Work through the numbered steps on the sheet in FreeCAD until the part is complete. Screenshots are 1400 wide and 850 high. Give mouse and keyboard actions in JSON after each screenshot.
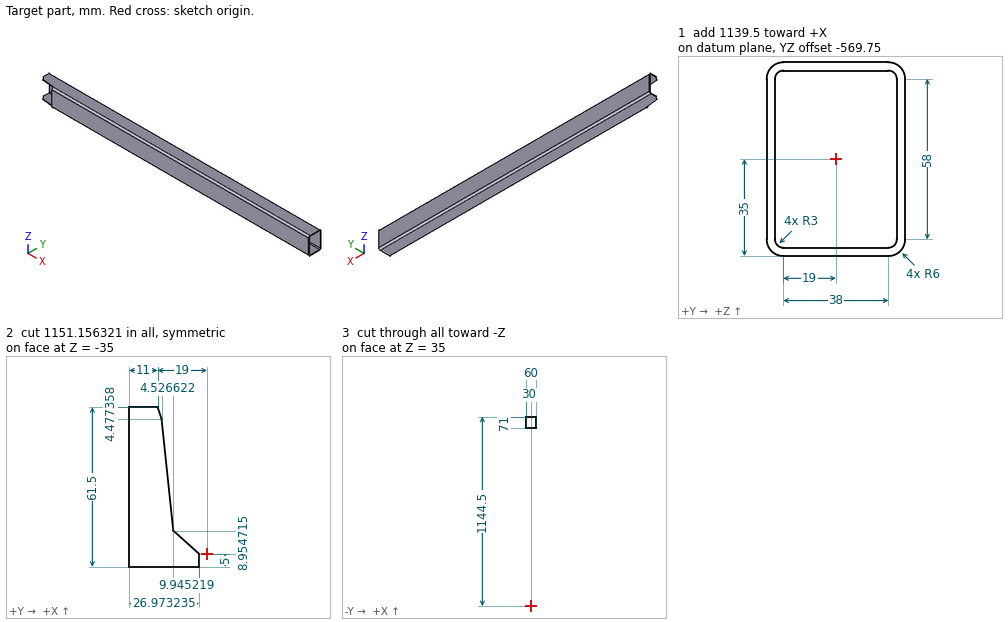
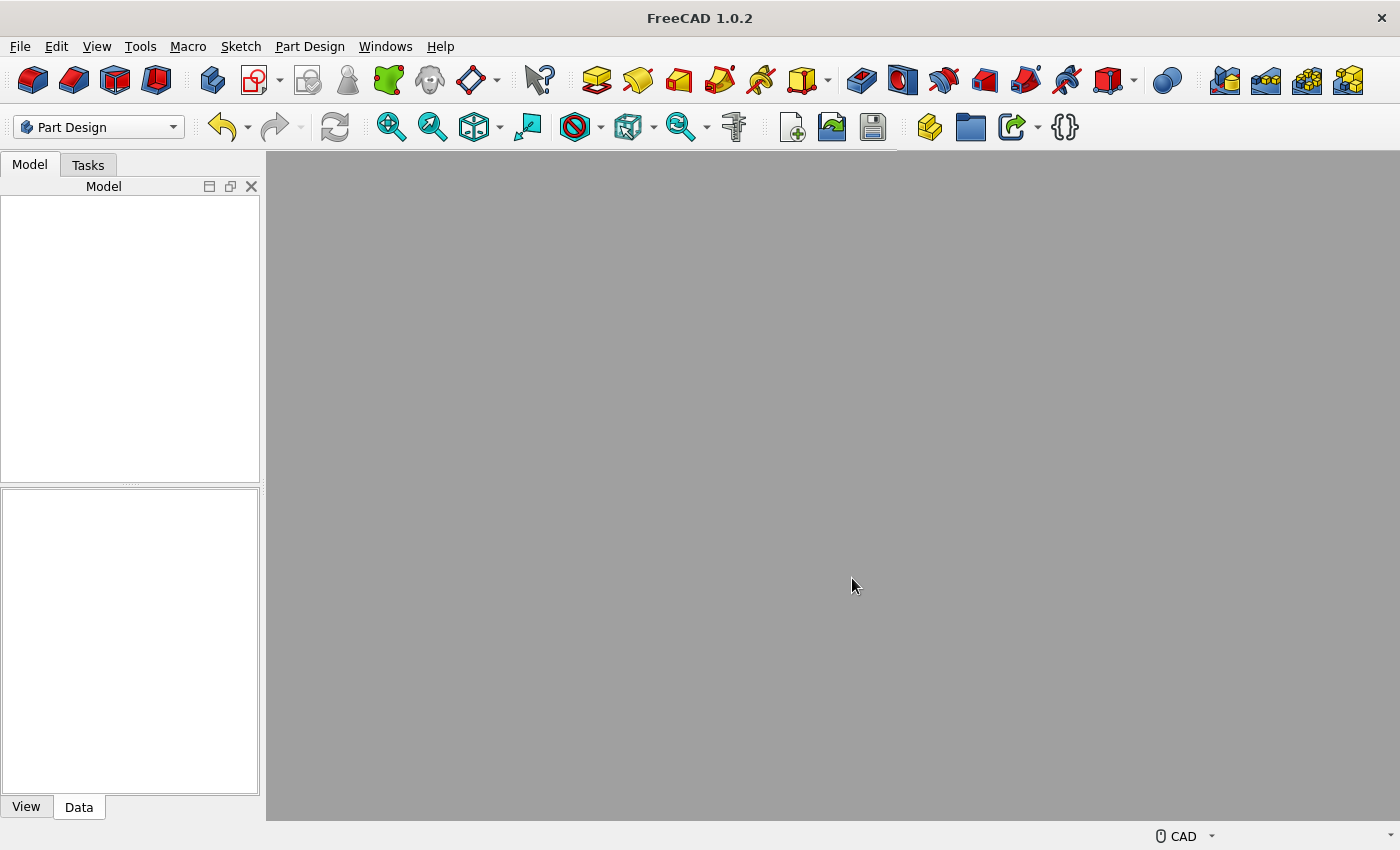
{"action": "key", "text": "ctrl+n"}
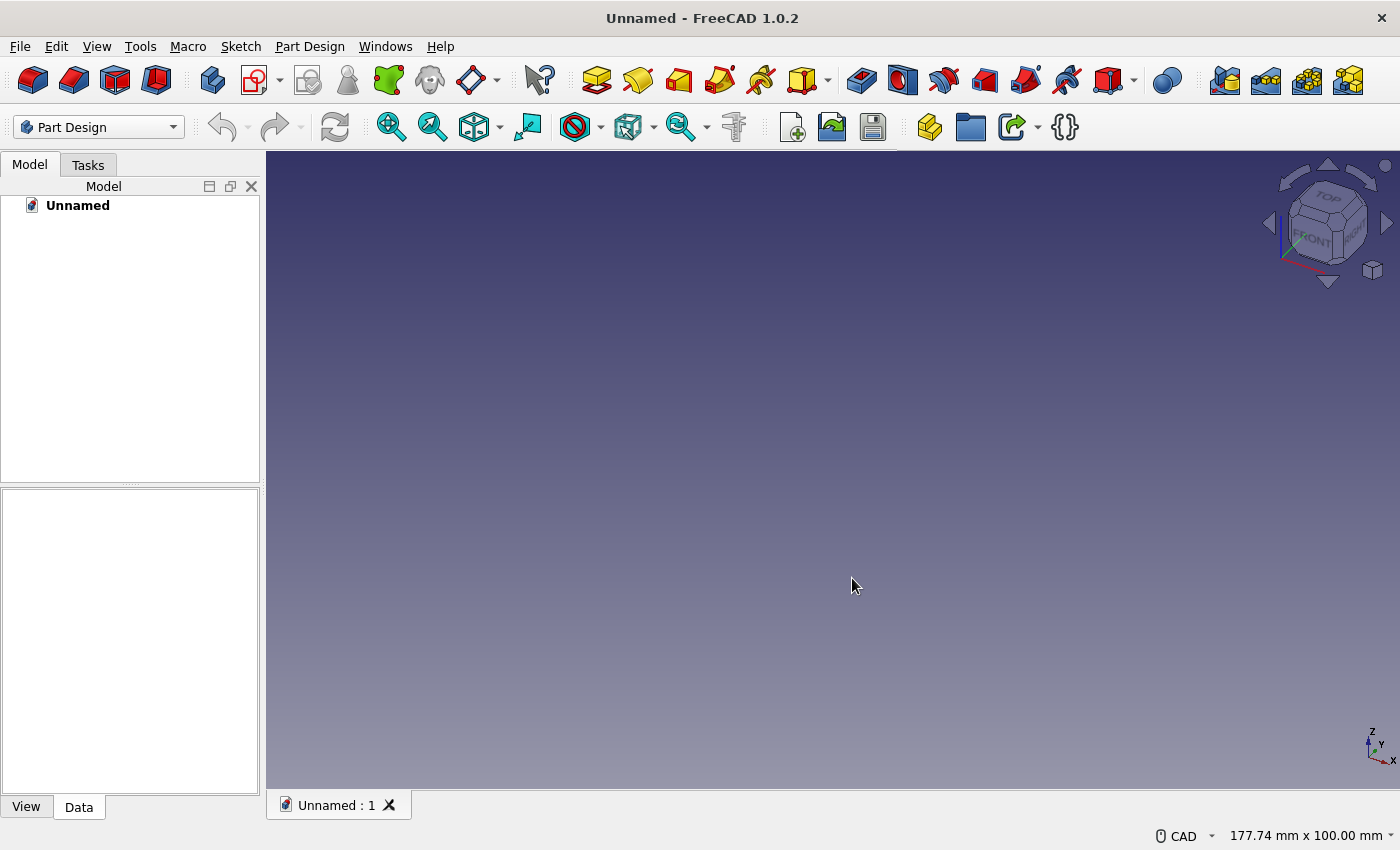
{"action": "left_click", "coordinate": [213, 80]}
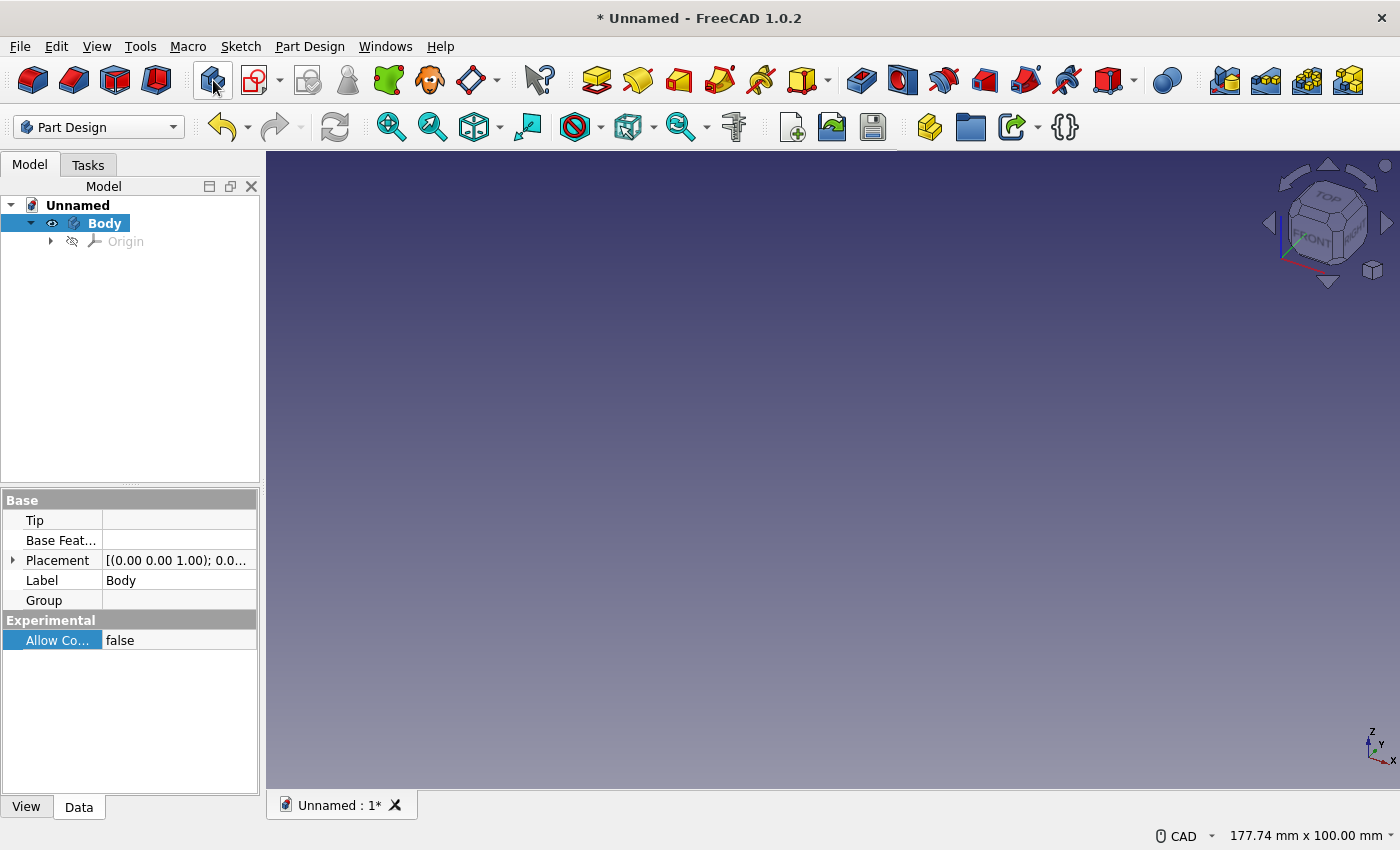
{"action": "left_click", "coordinate": [51, 241]}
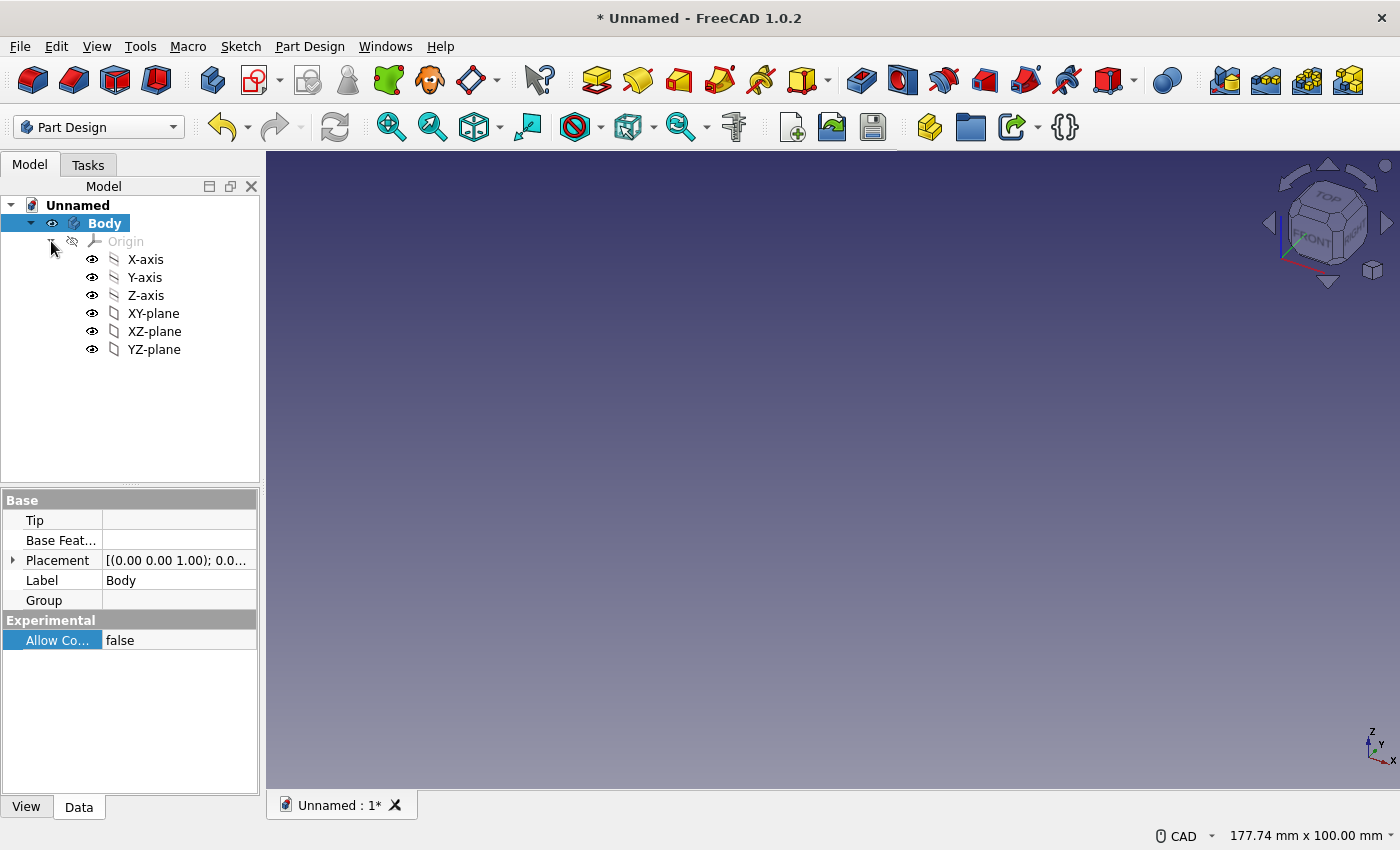
{"action": "left_click", "coordinate": [137, 349]}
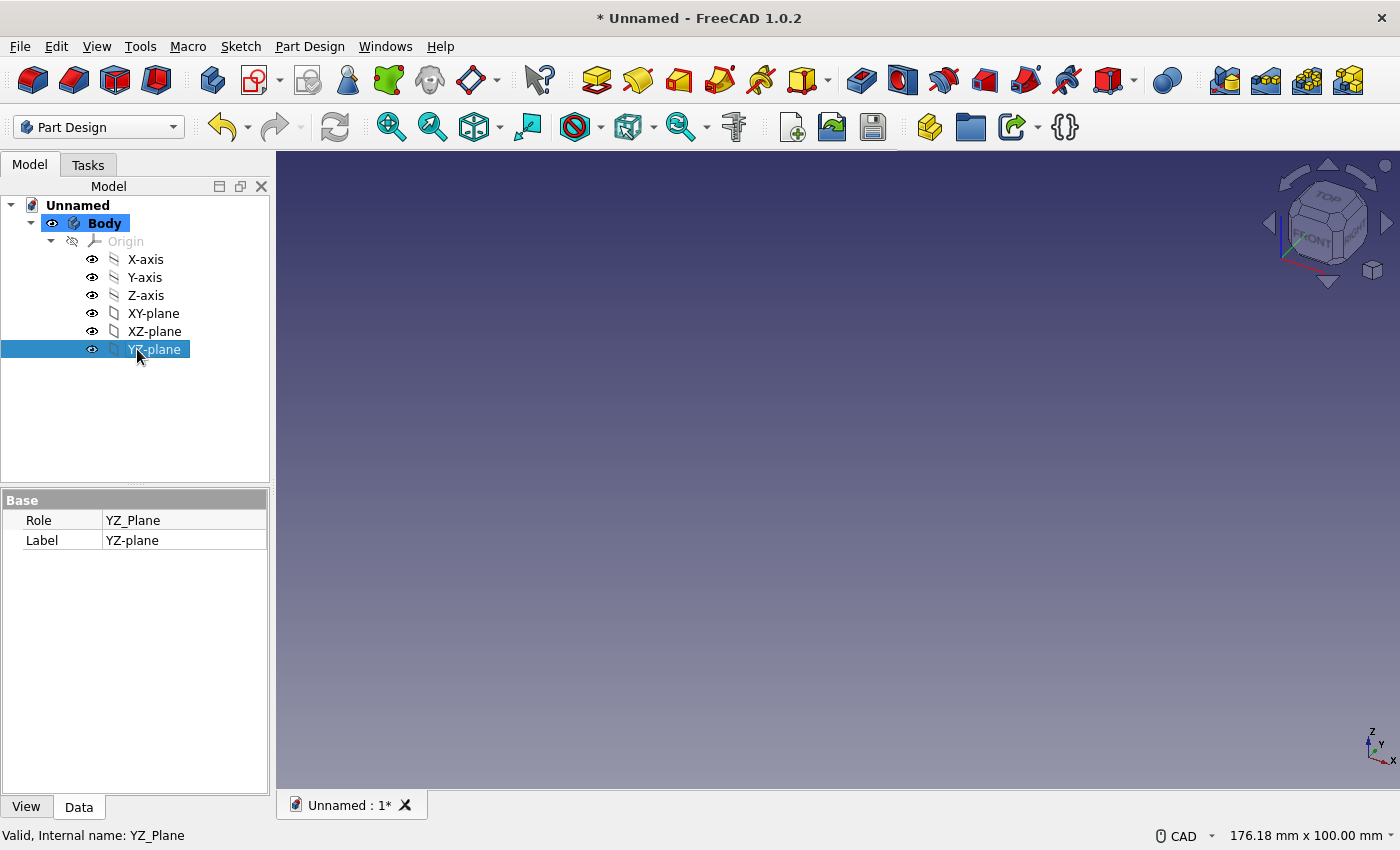
{"action": "left_click", "coordinate": [470, 80]}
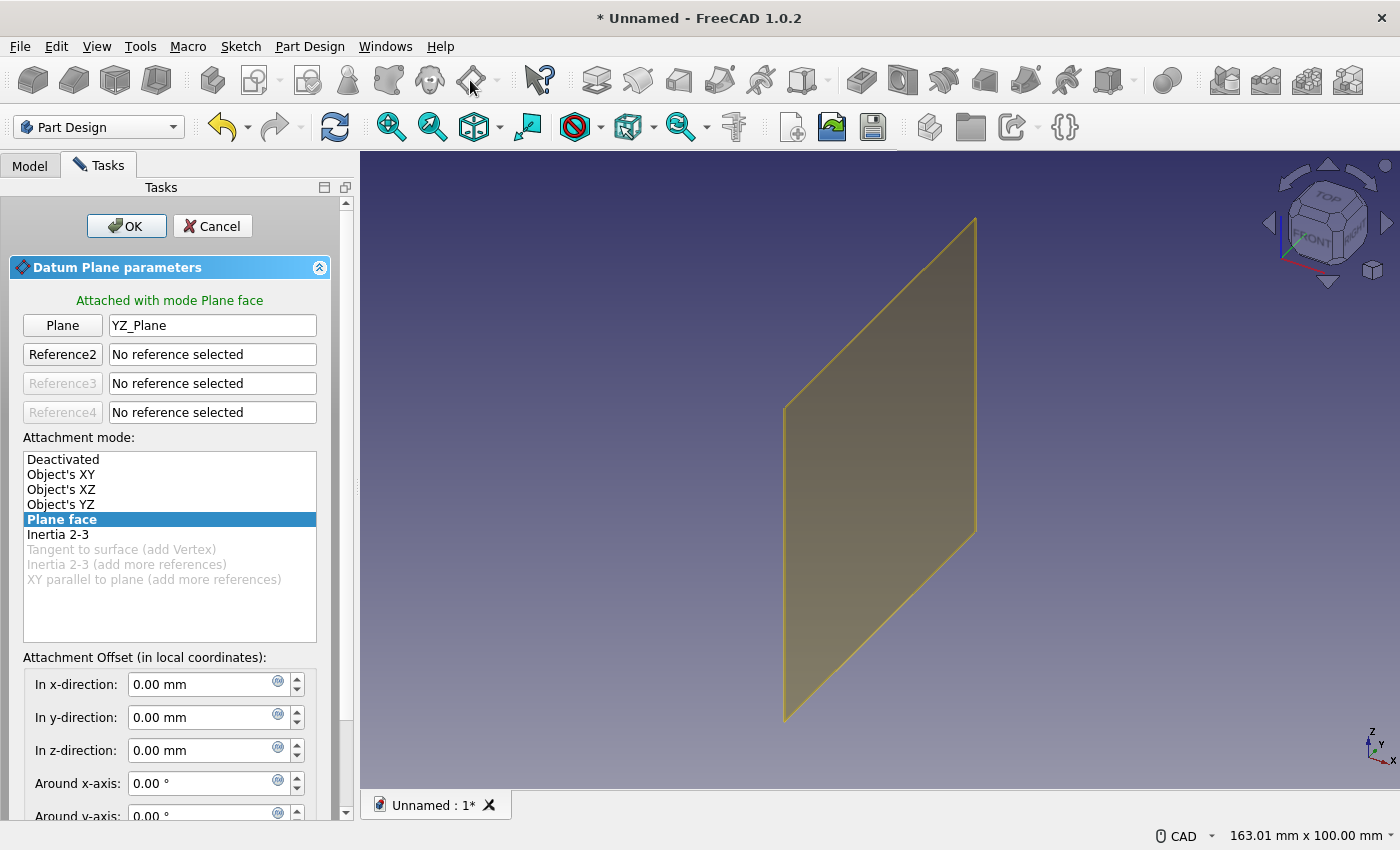
{"action": "triple_click", "coordinate": [210, 750]}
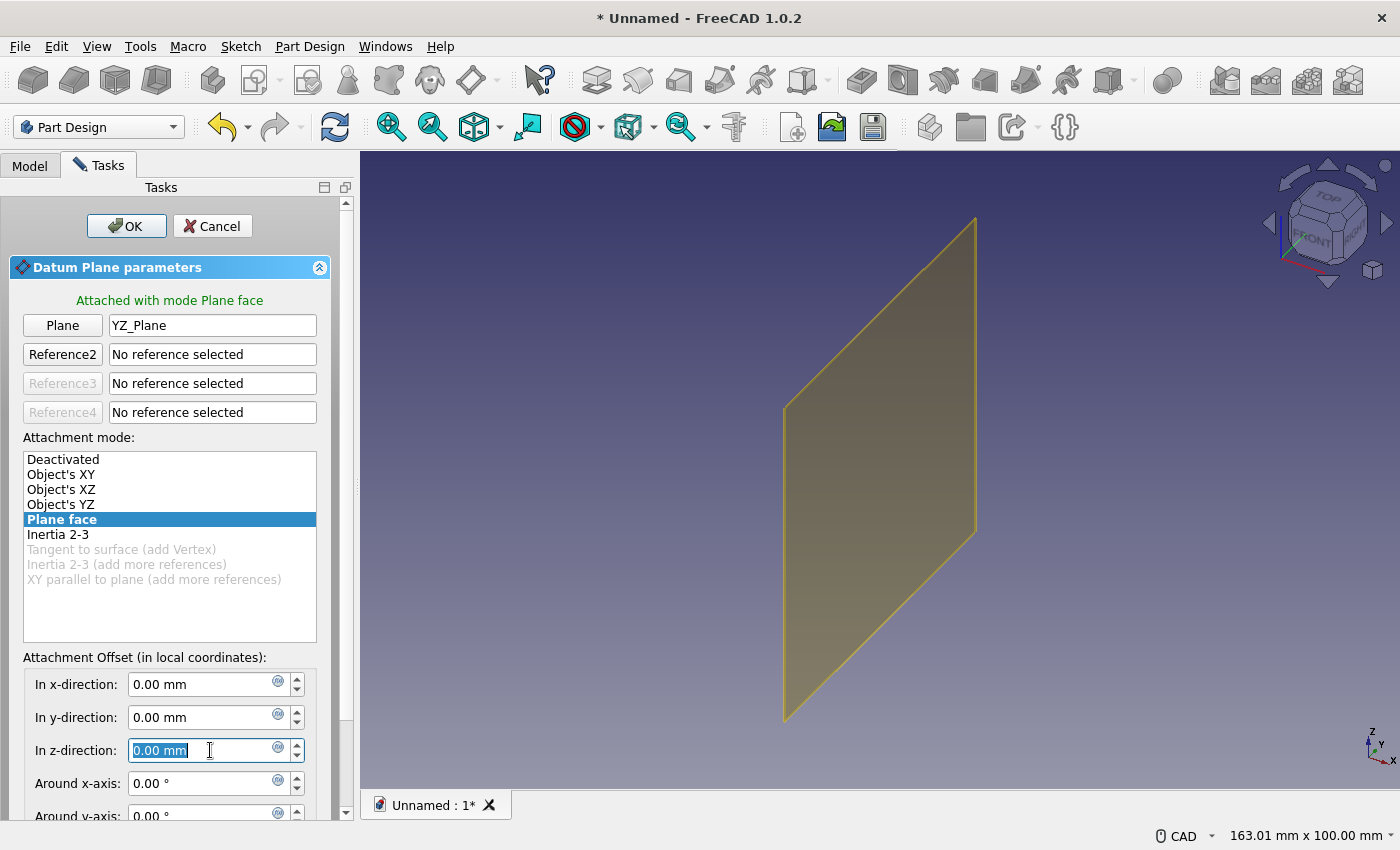
{"action": "type", "text": "-569.75"}
{"action": "key", "text": "Tab"}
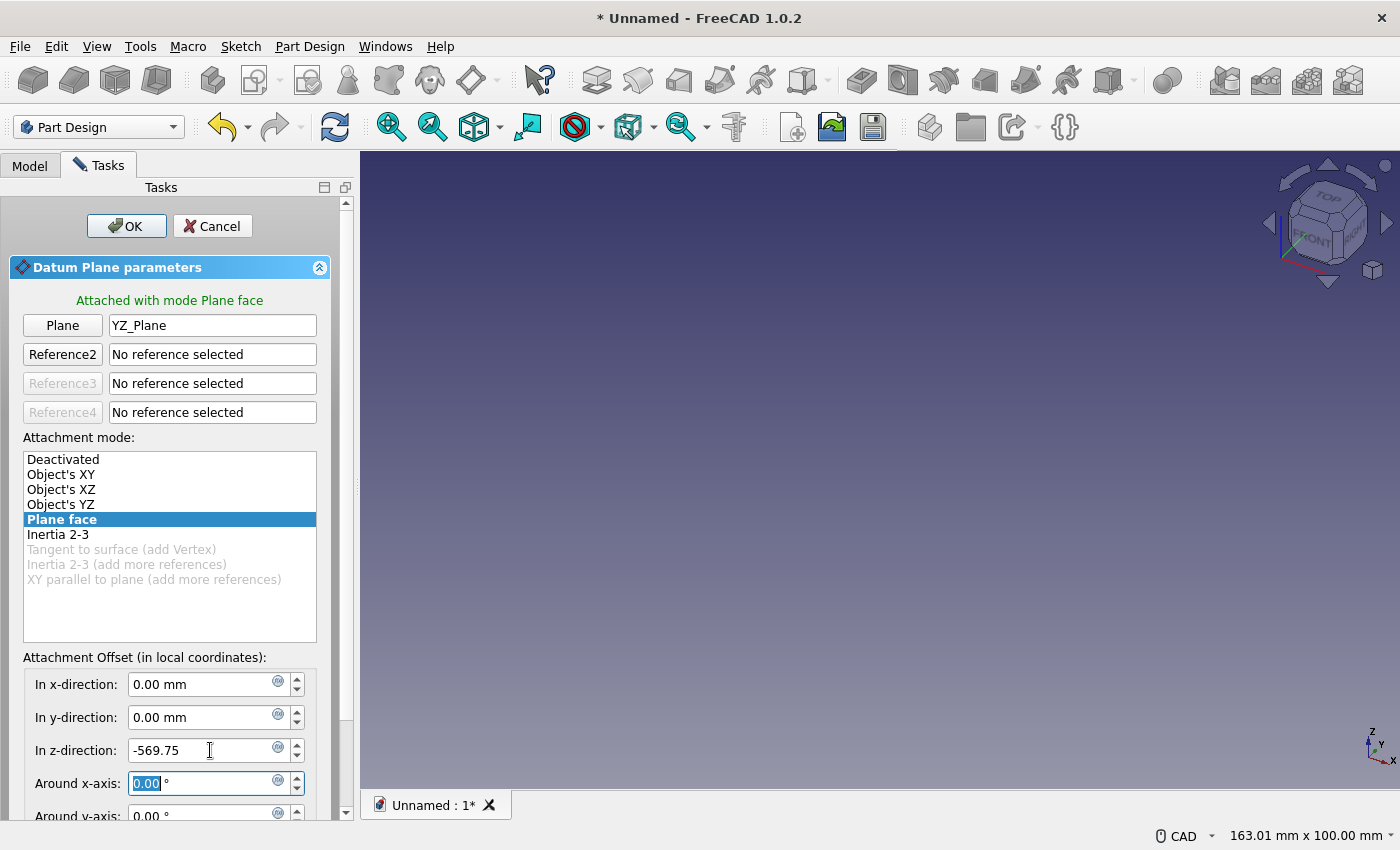
{"action": "left_click", "coordinate": [127, 226]}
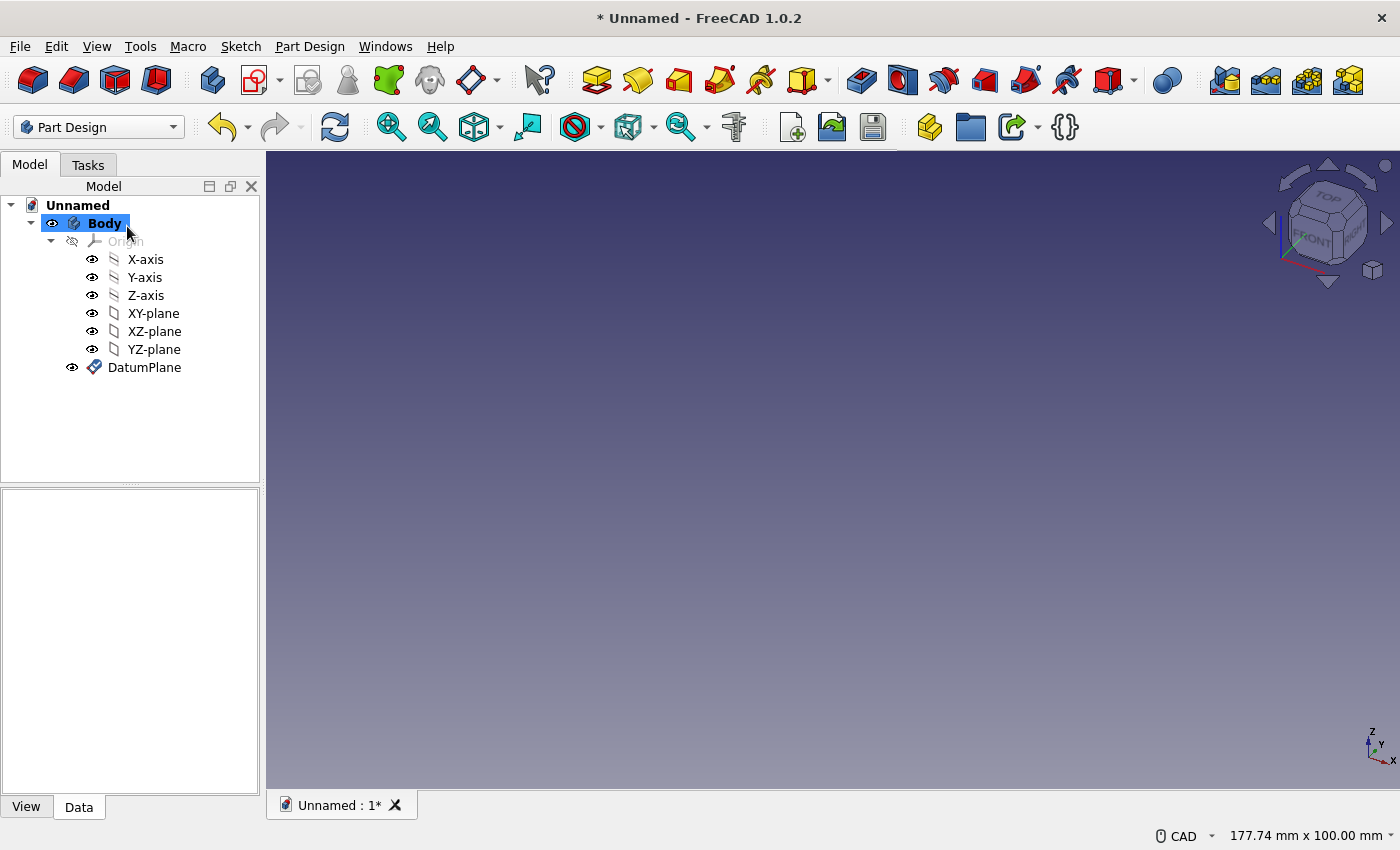
{"action": "left_click", "coordinate": [117, 367]}